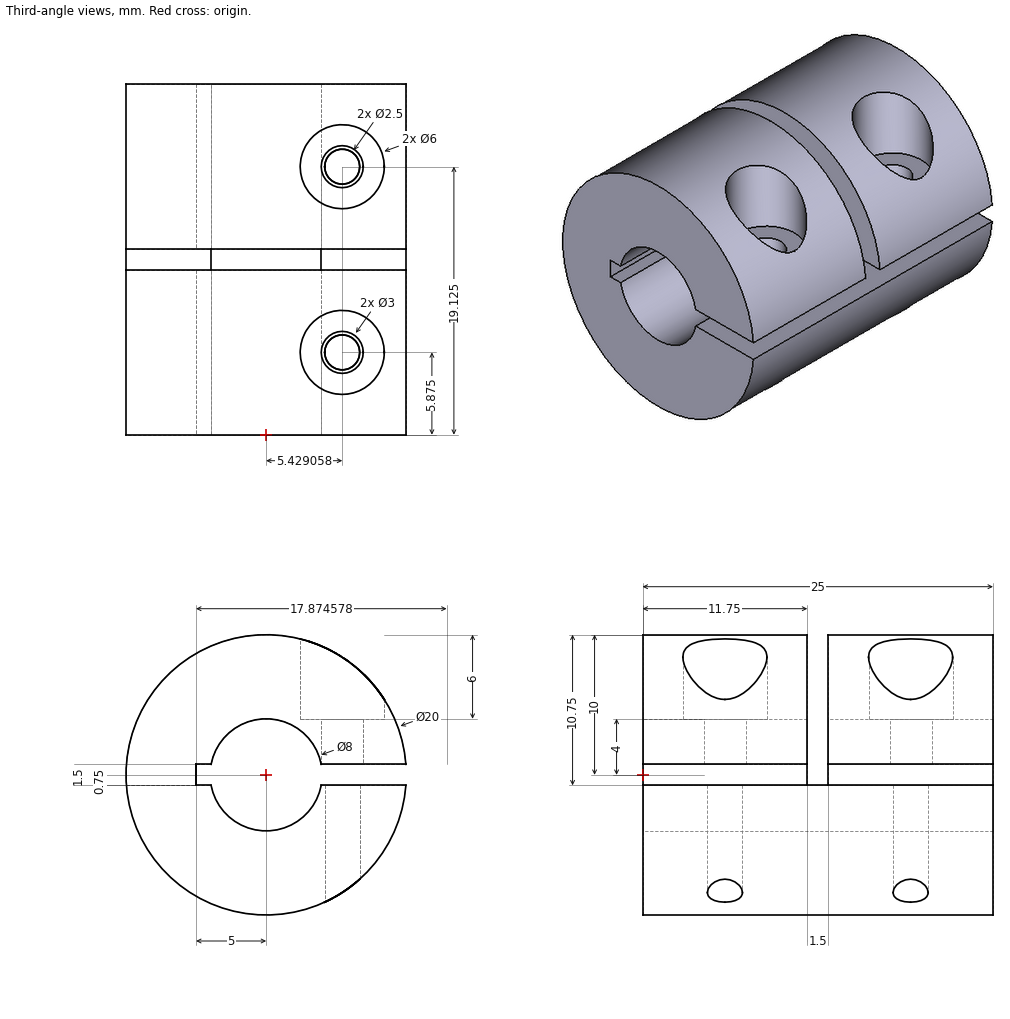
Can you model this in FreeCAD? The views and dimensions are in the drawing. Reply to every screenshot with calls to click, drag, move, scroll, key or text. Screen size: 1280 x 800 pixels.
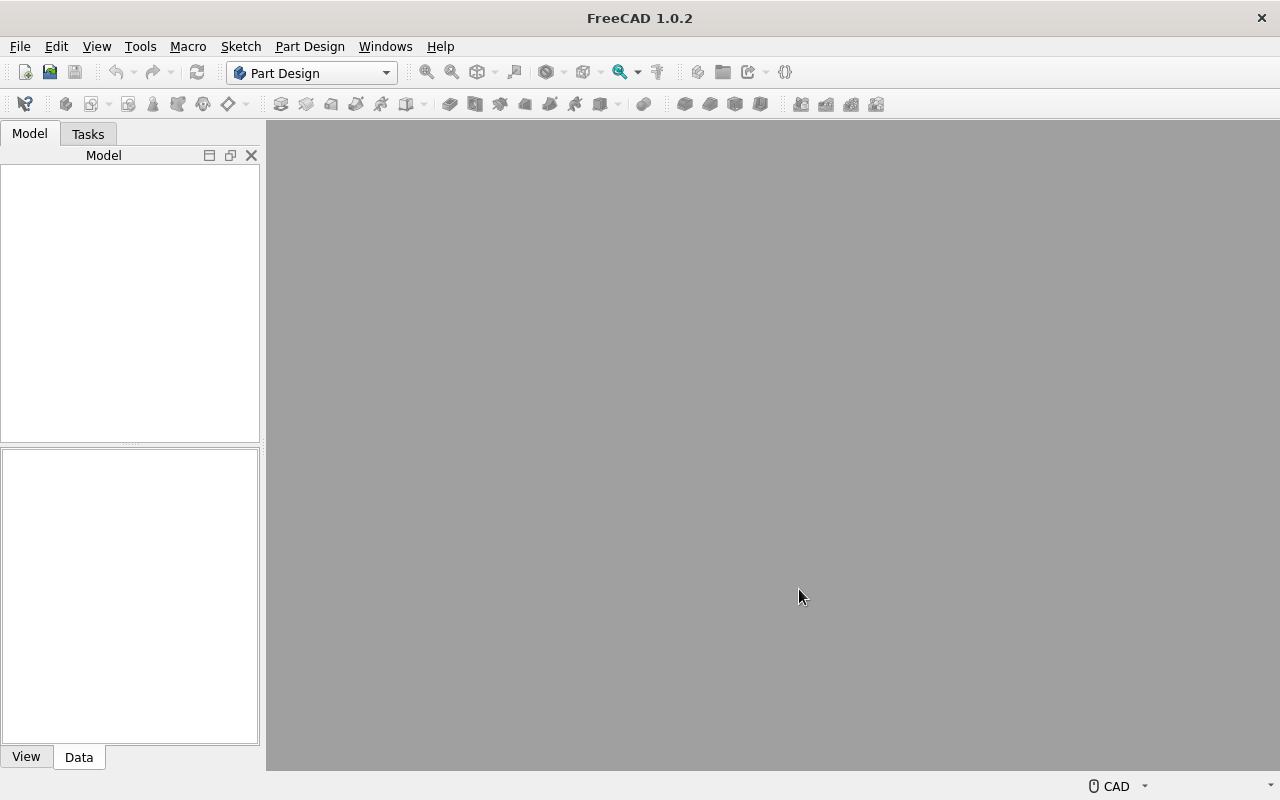
click(25, 72)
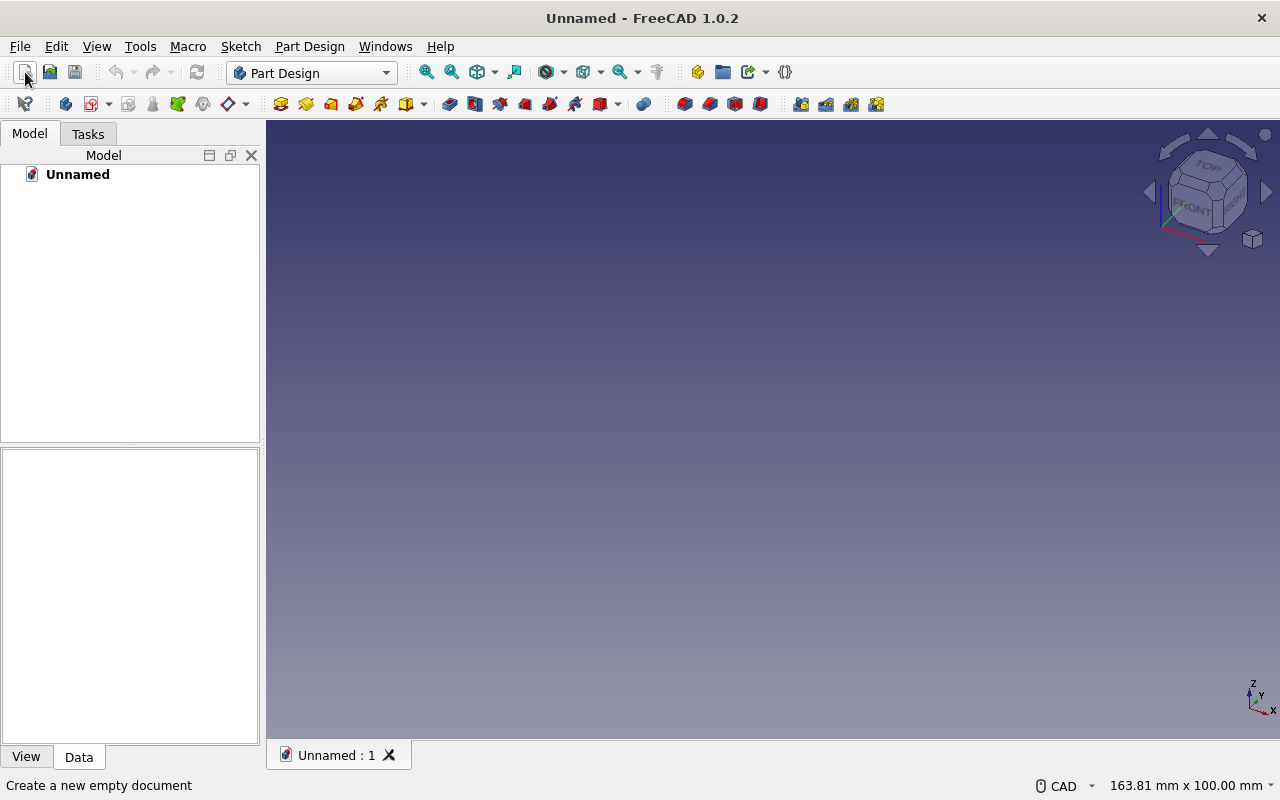
click(90, 104)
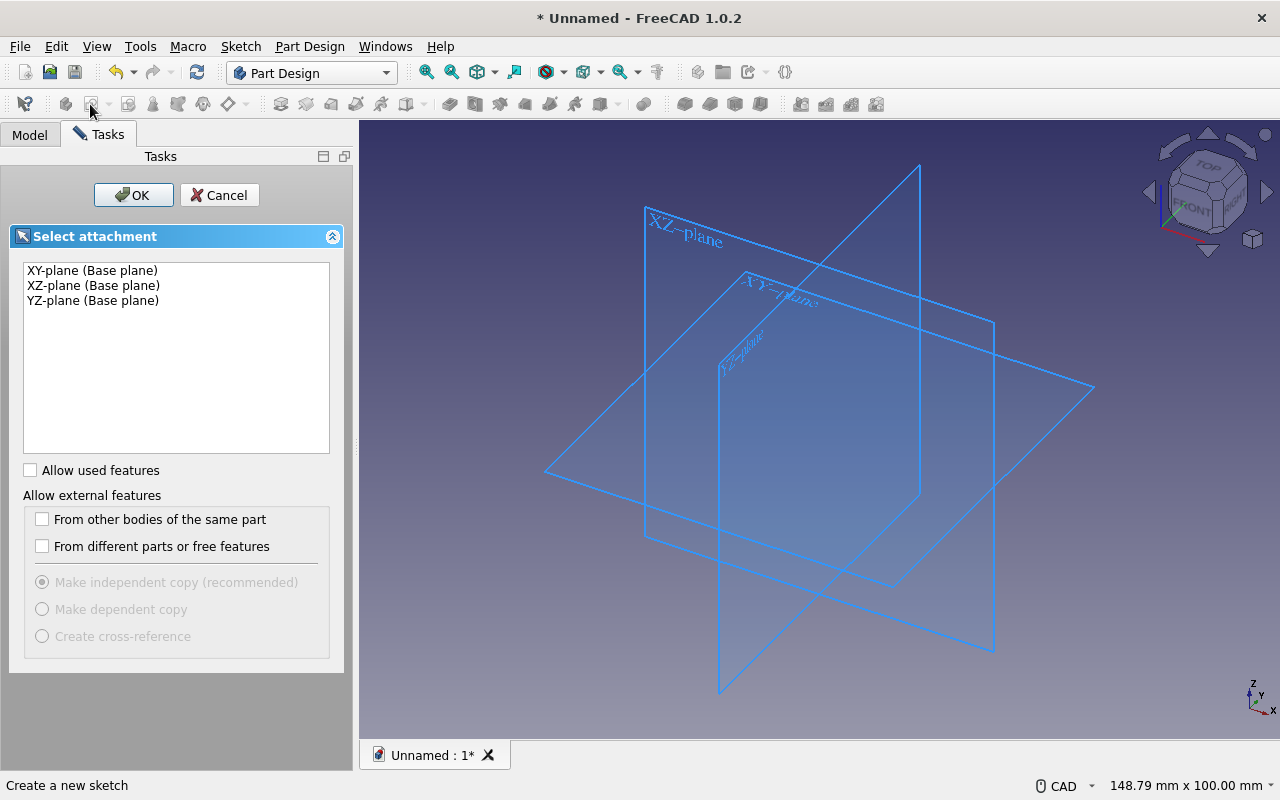
click(84, 286)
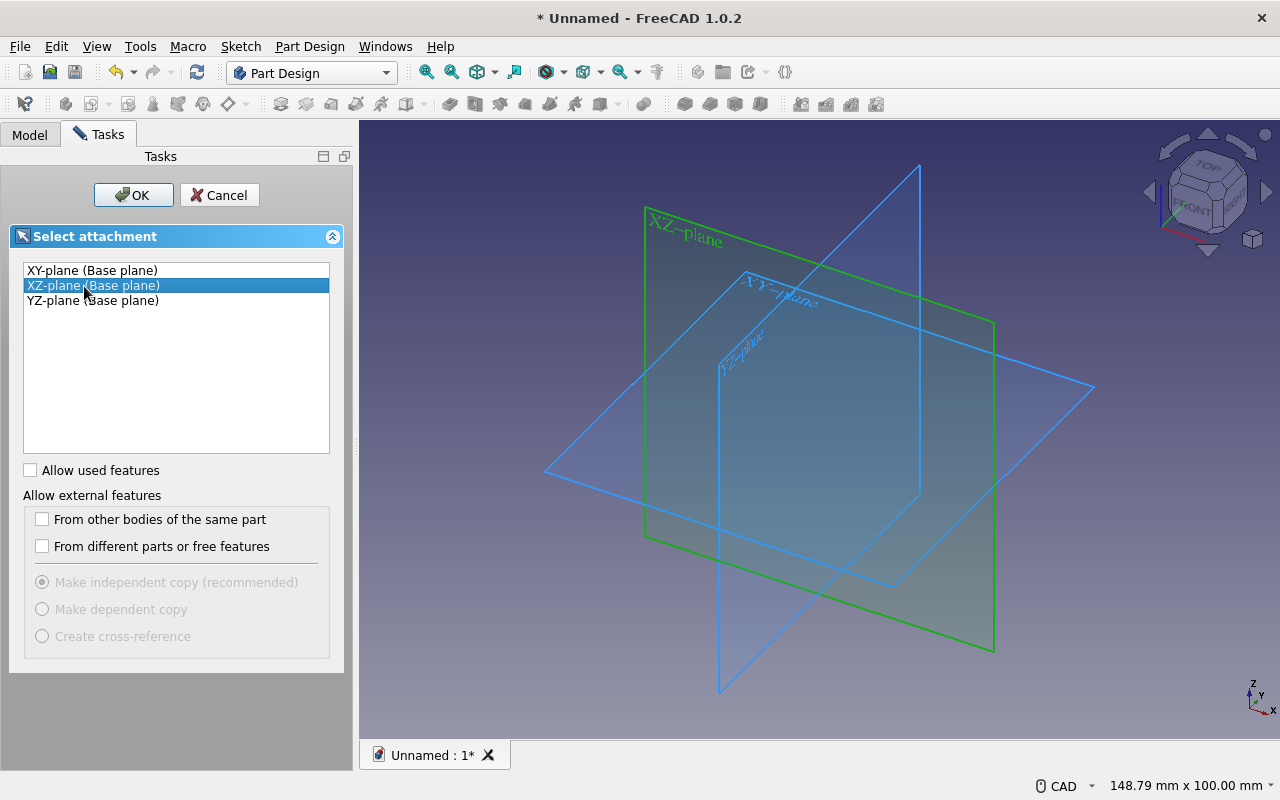
click(134, 195)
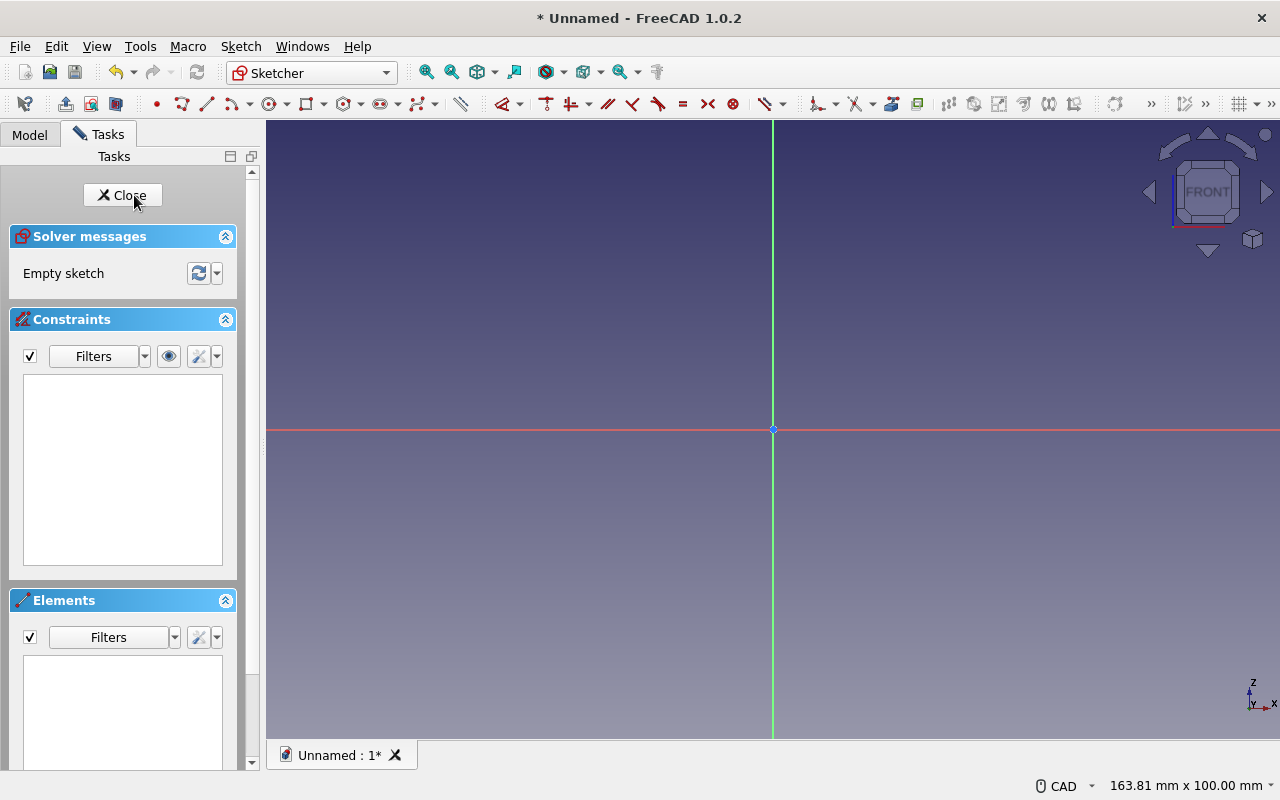
scroll(803, 430, up, 6)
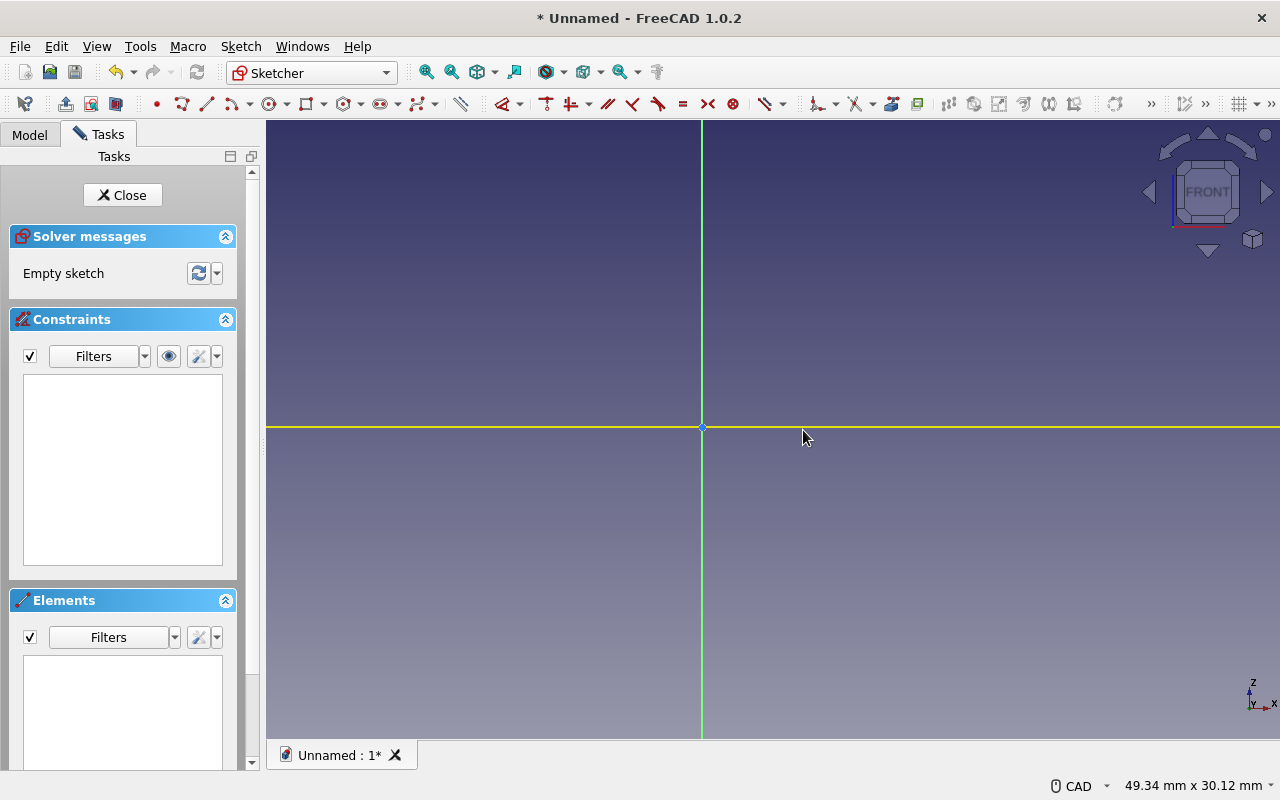
click(268, 104)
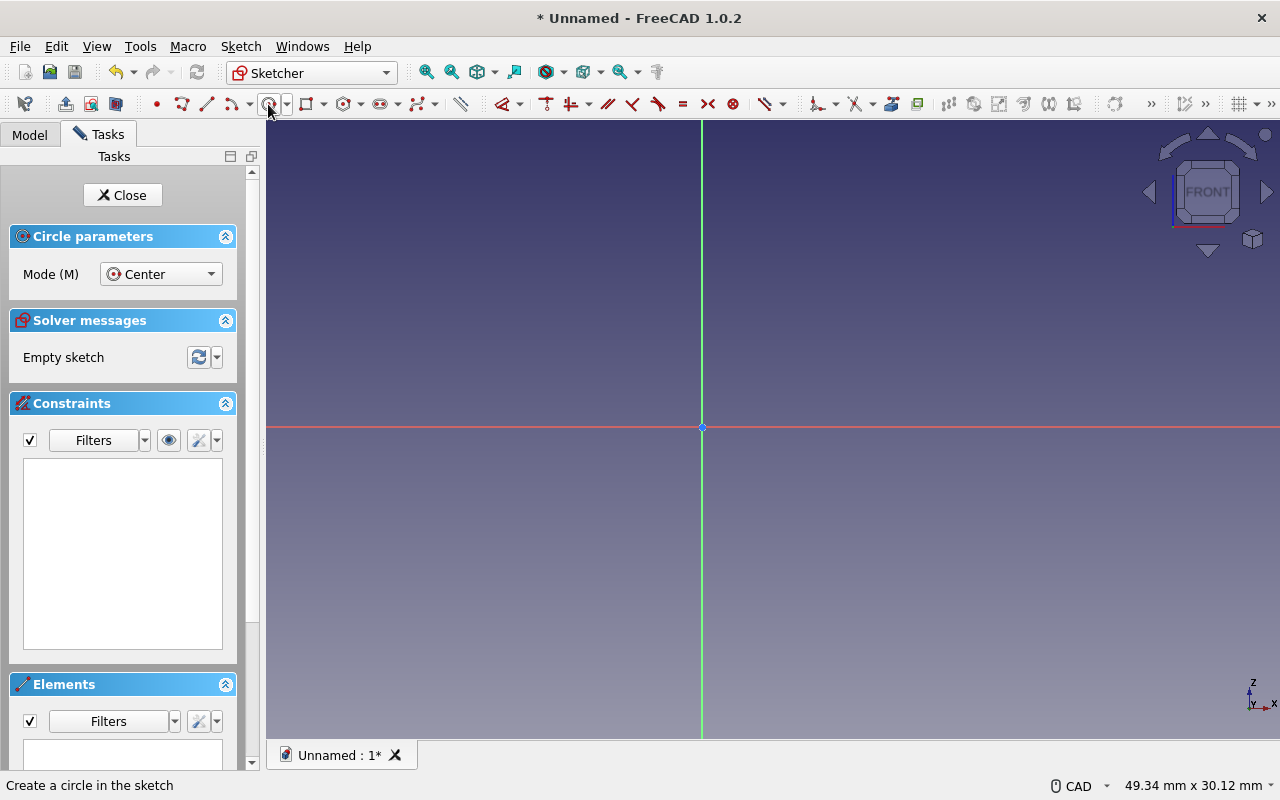
click(702, 427)
click(847, 282)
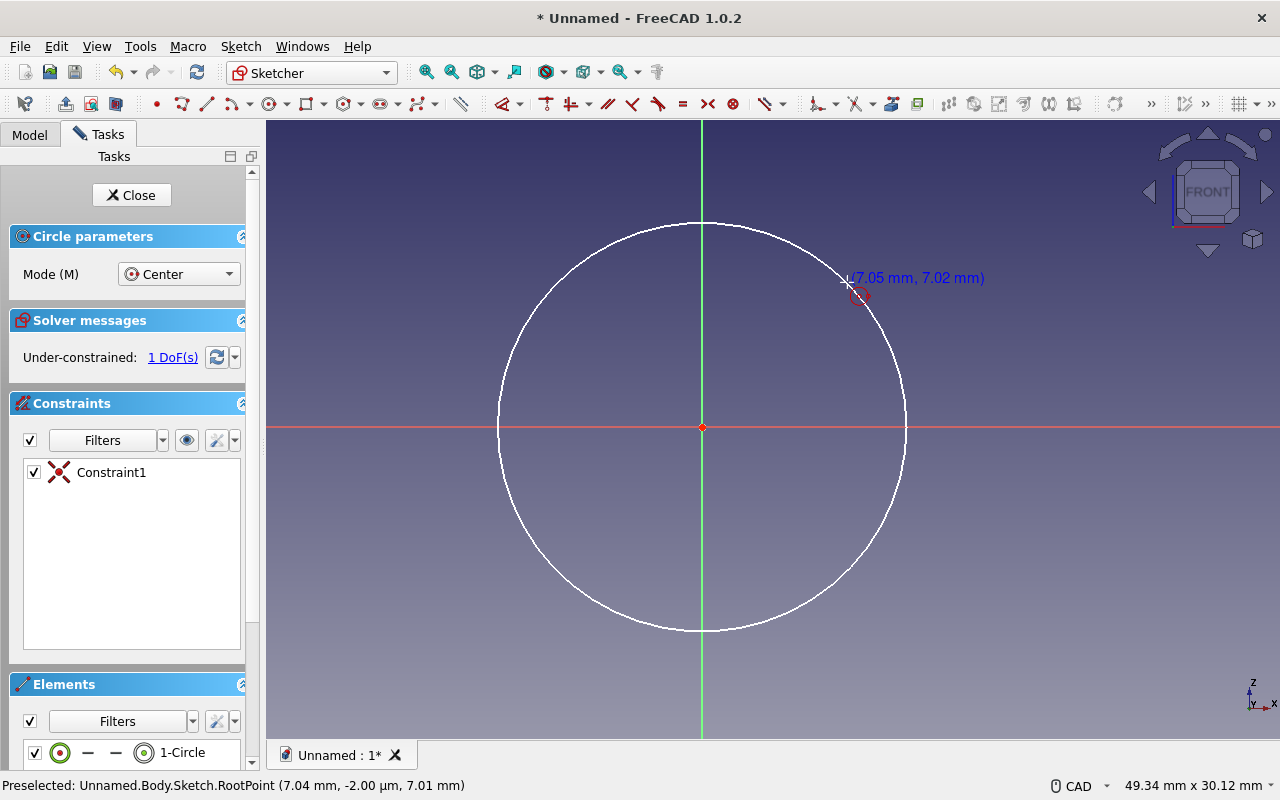
click(702, 427)
click(760, 369)
key(Escape)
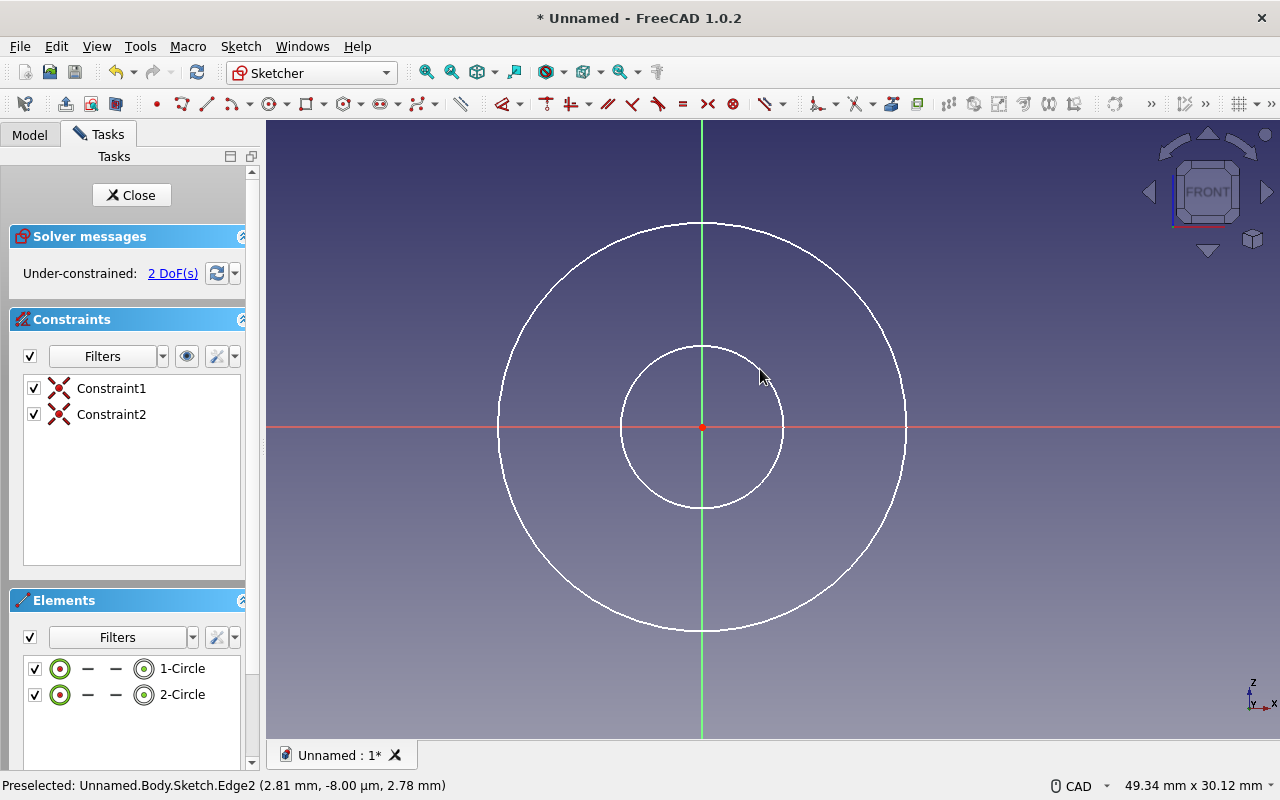
click(846, 282)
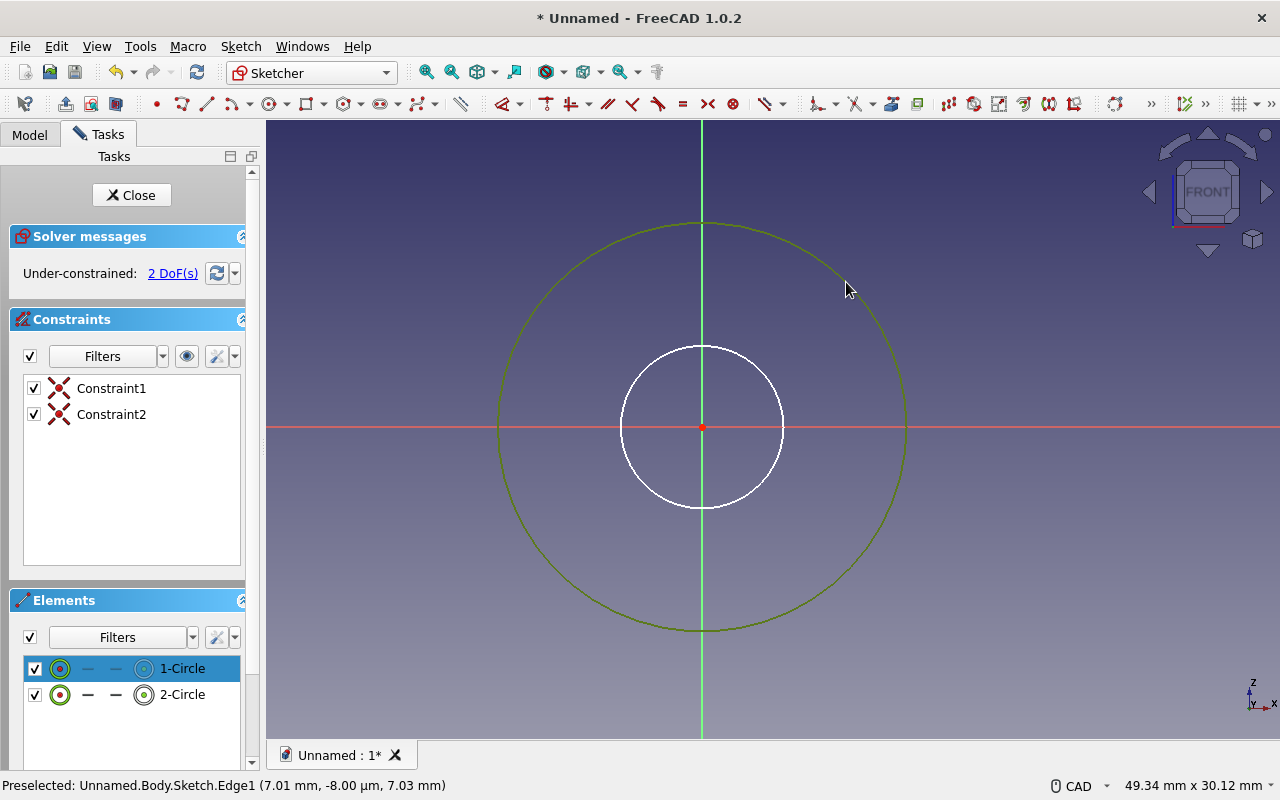
key(k)
key(o)